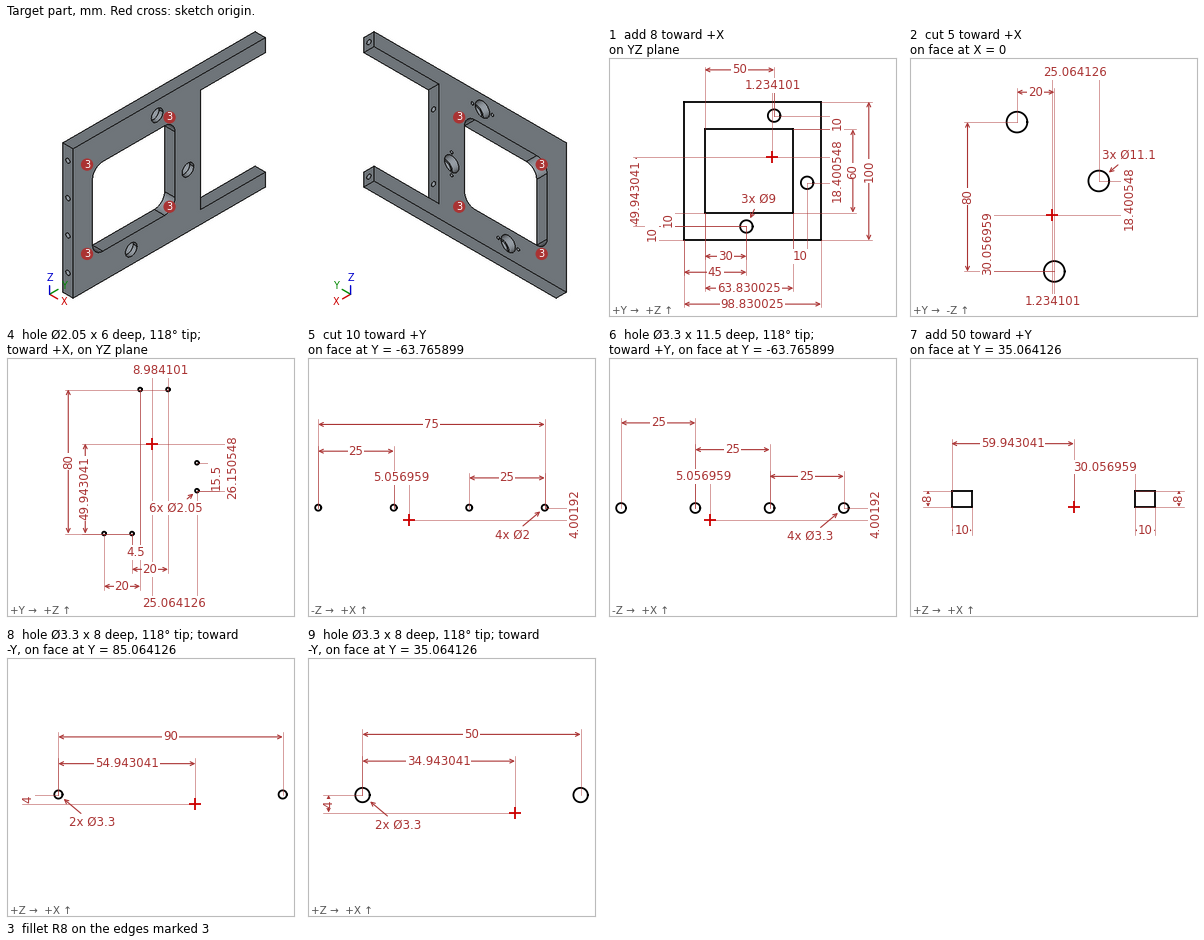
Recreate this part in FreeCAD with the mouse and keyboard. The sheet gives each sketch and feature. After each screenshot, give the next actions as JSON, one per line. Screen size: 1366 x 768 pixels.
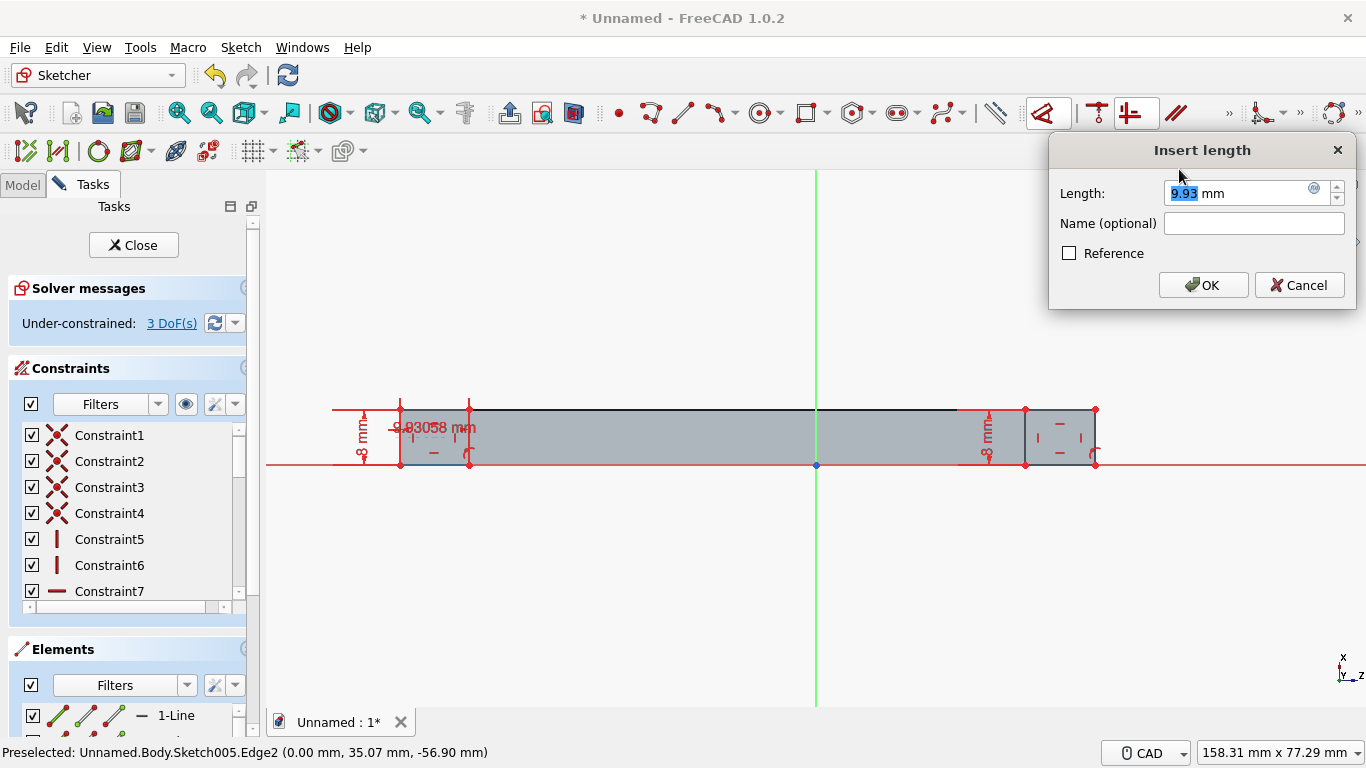
{"action": "type", "text": "10"}
{"action": "key", "text": "Return"}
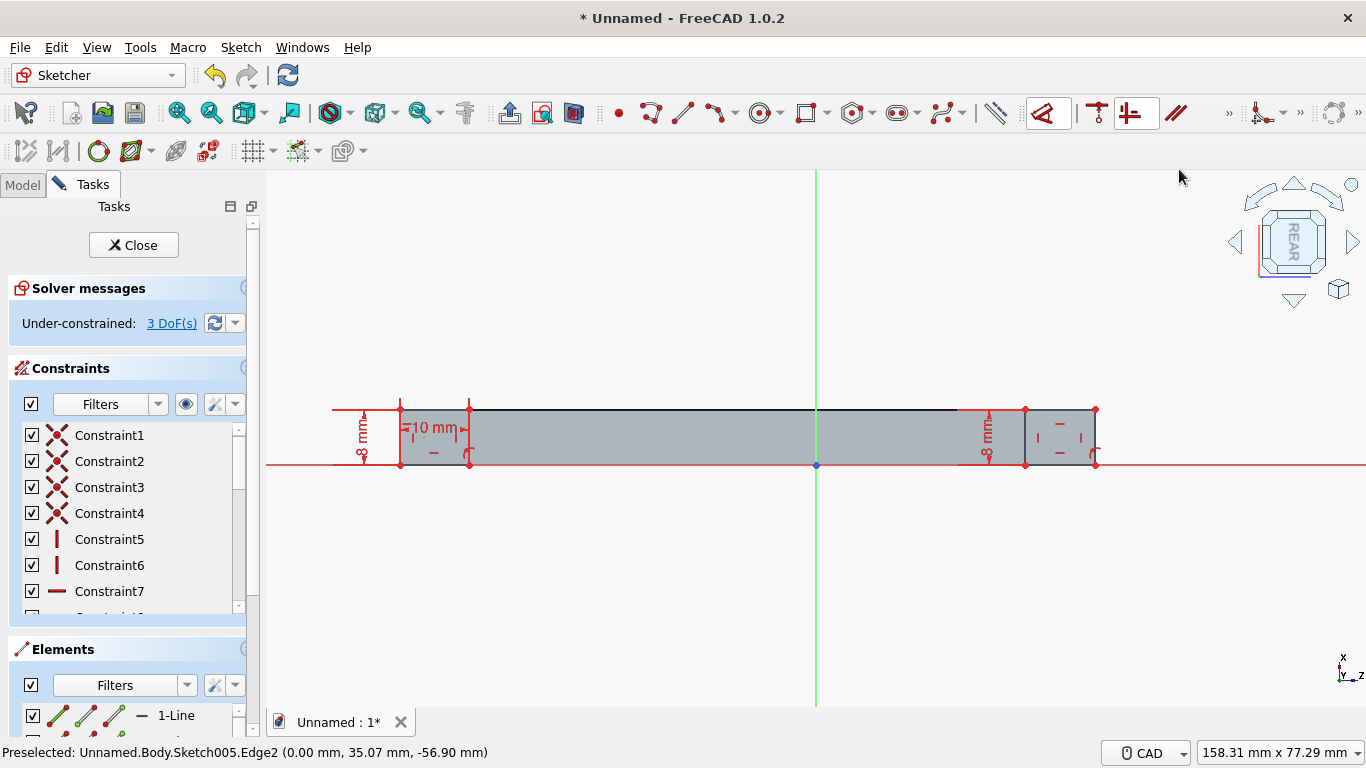
{"action": "left_click", "coordinate": [1046, 465]}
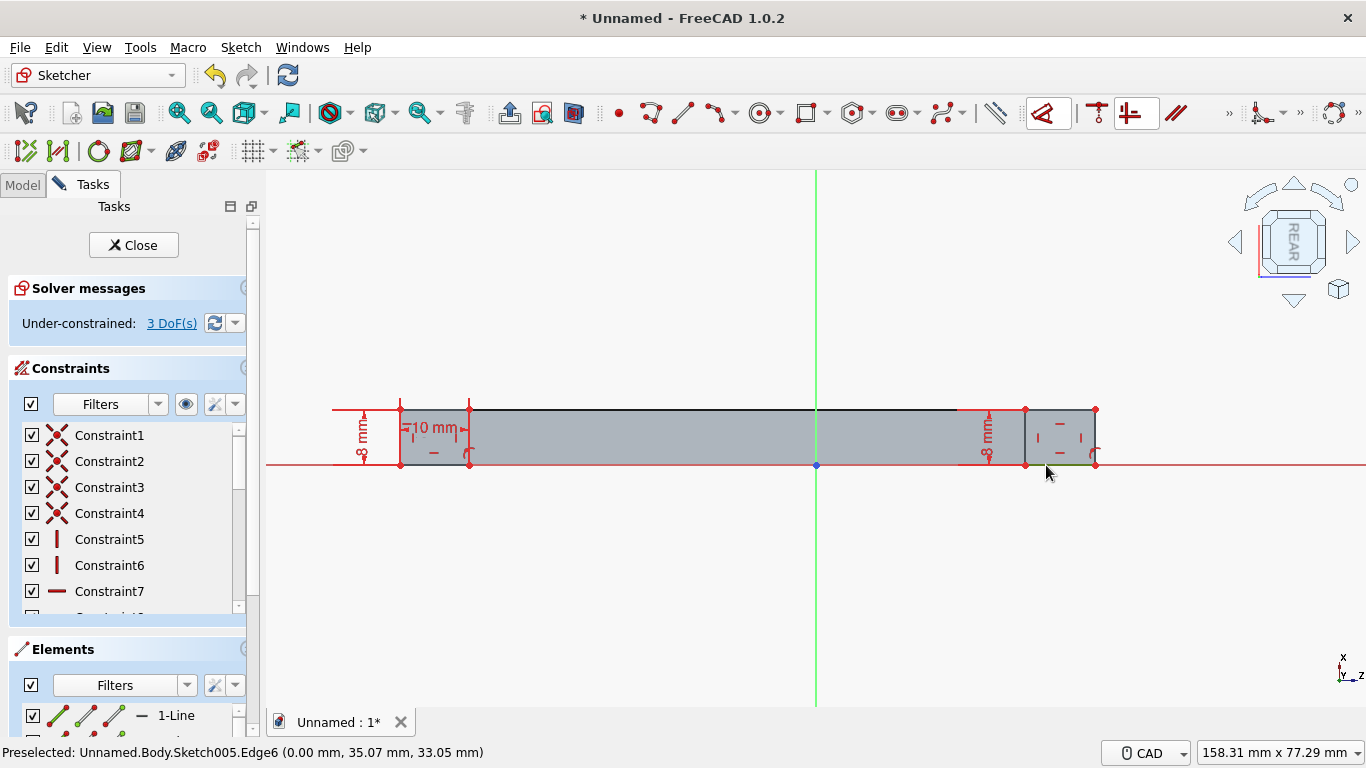
{"action": "key", "text": "l"}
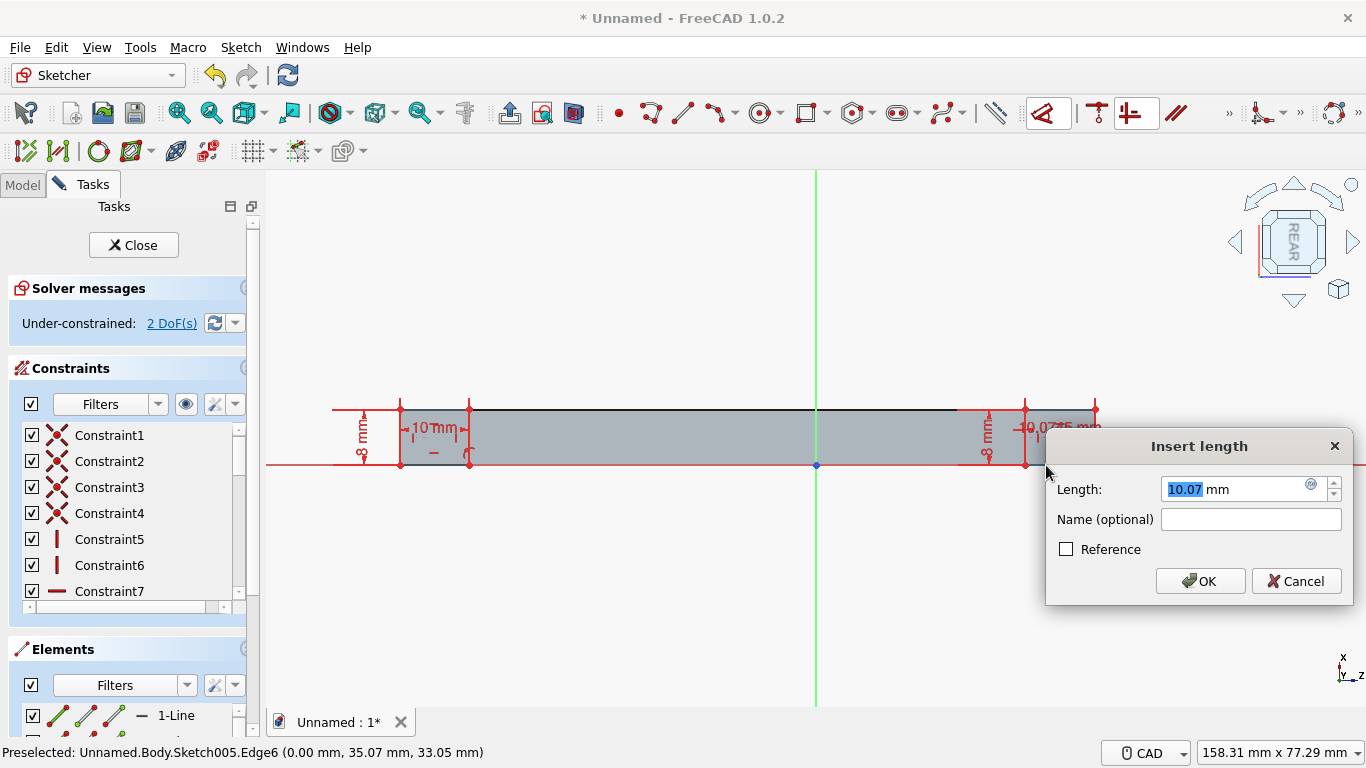
{"action": "type", "text": "10"}
{"action": "key", "text": "Return"}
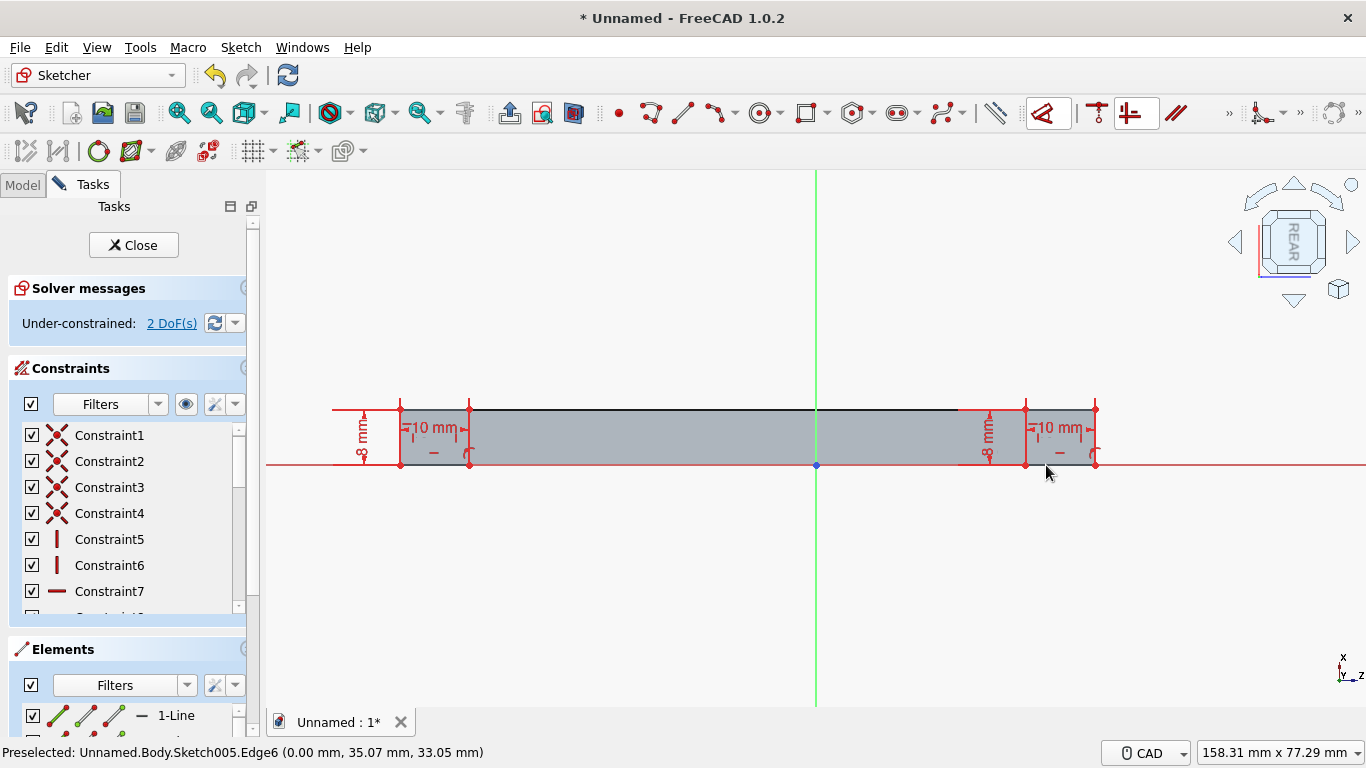
{"action": "left_click", "coordinate": [400, 410]}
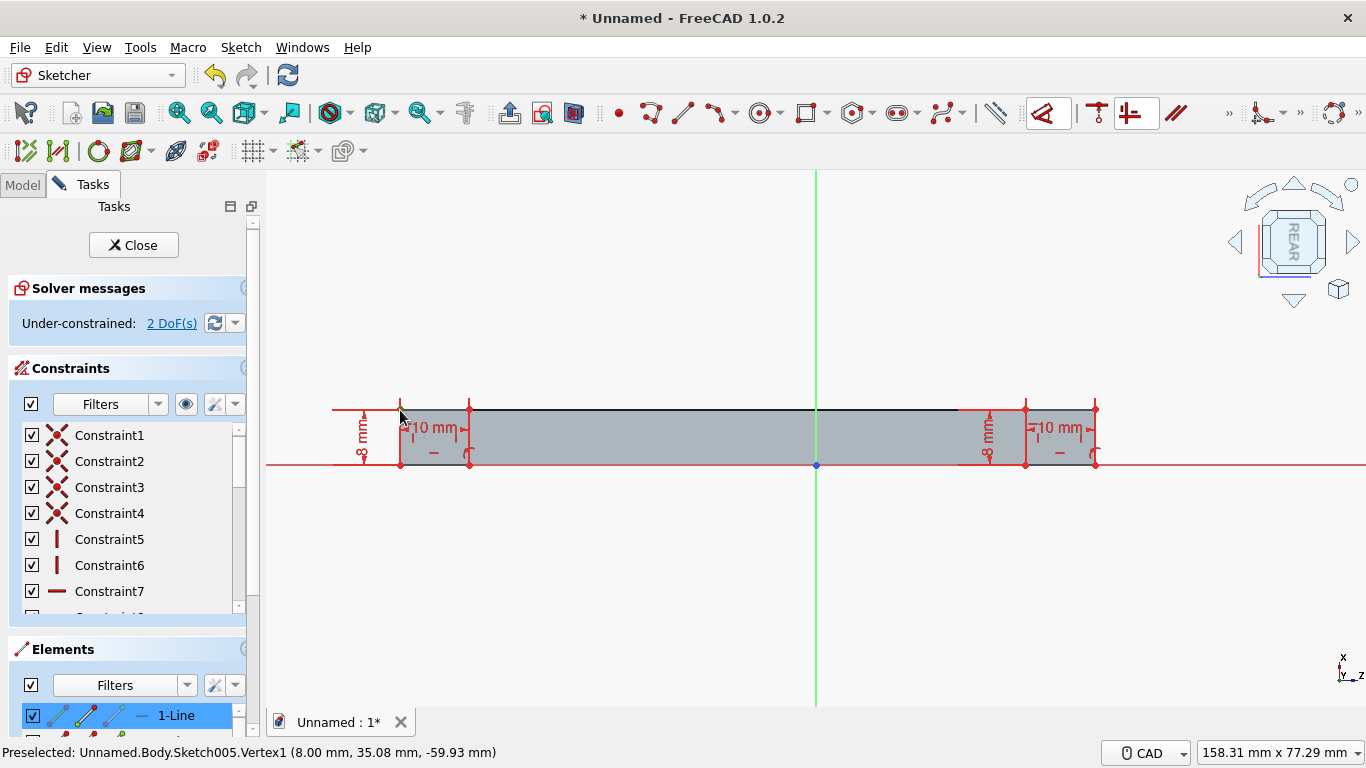
{"action": "key", "text": "l"}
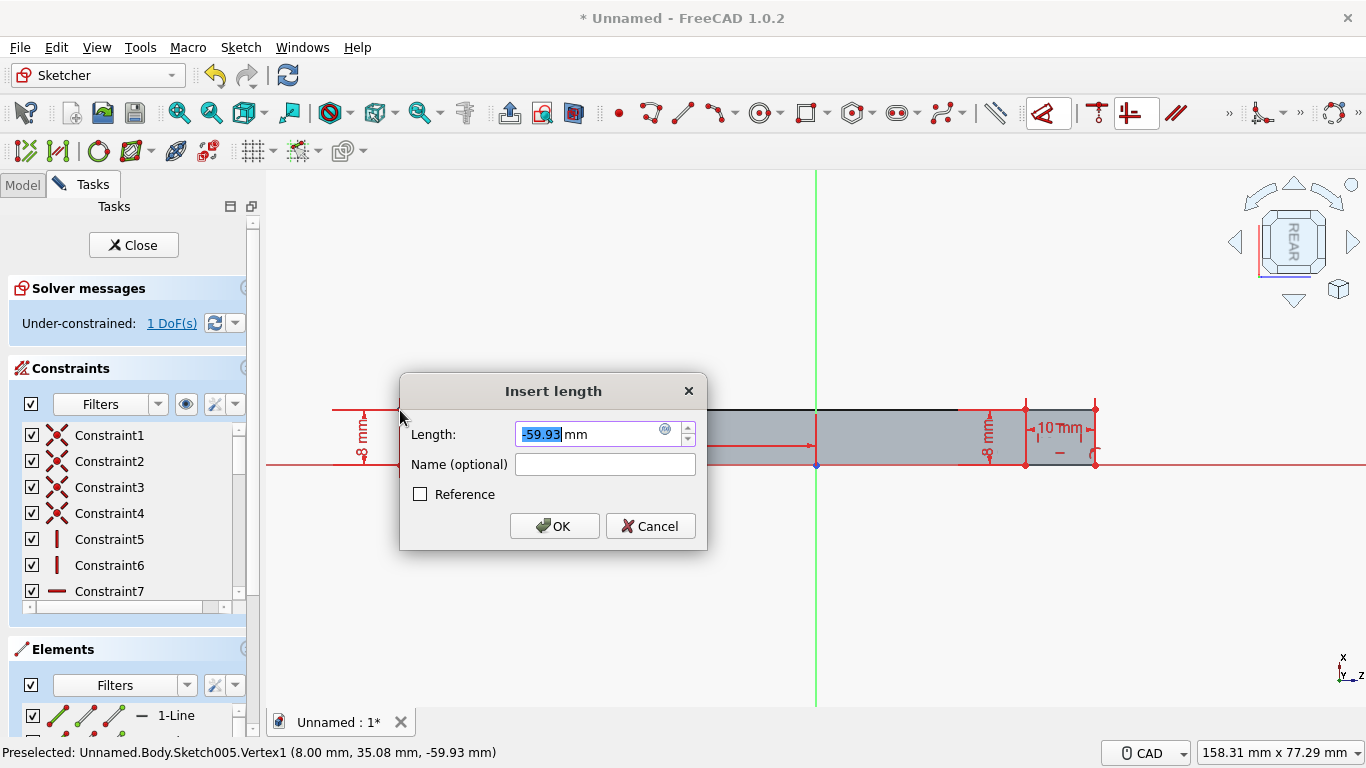
{"action": "type", "text": "-59.943041"}
{"action": "key", "text": "Return"}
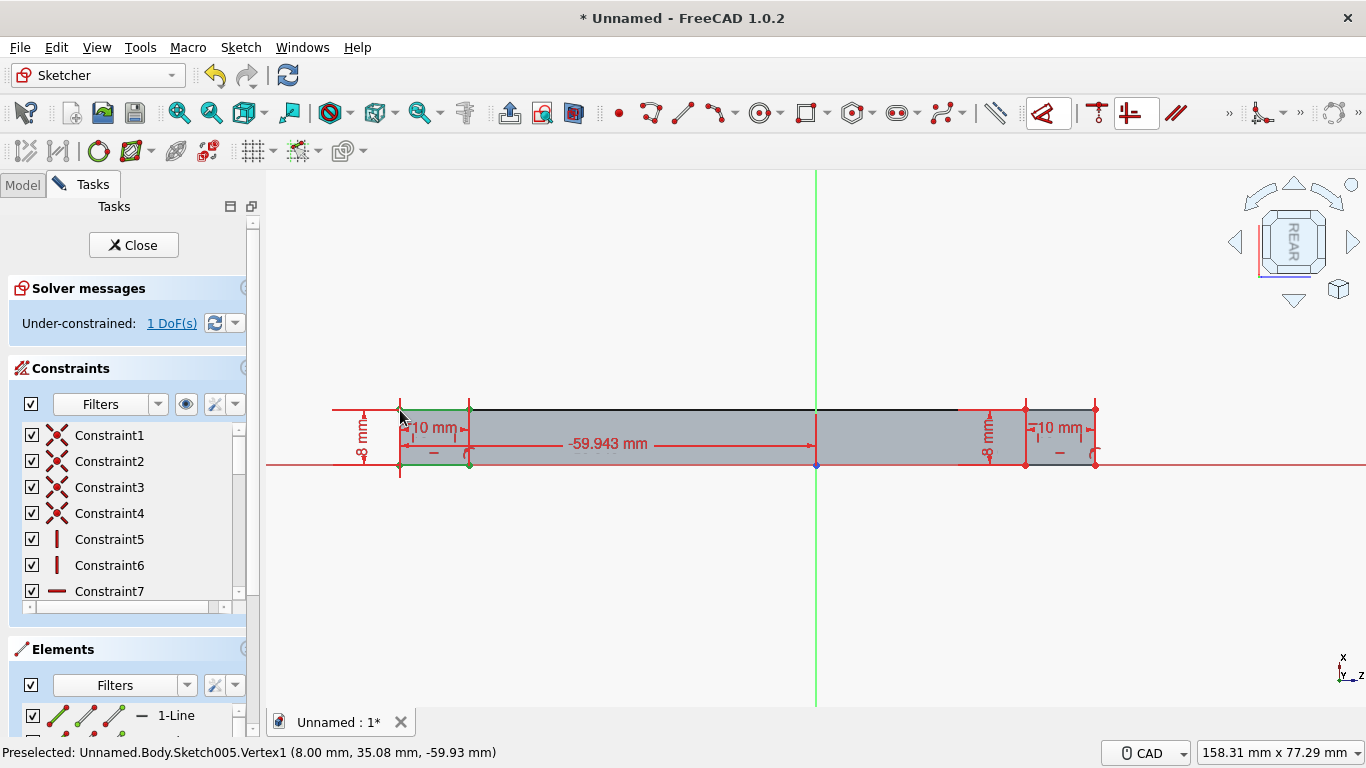
{"action": "left_click", "coordinate": [1026, 410]}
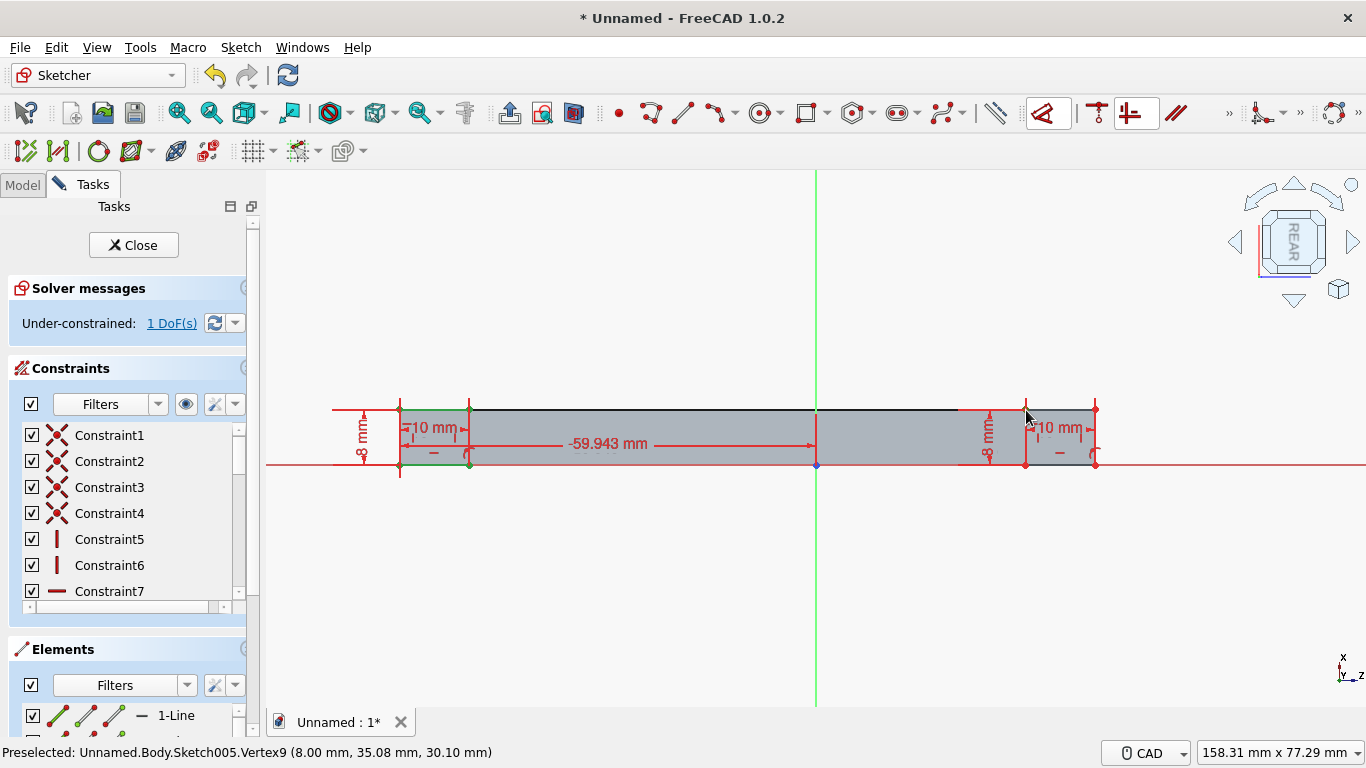
{"action": "left_click", "coordinate": [1066, 114]}